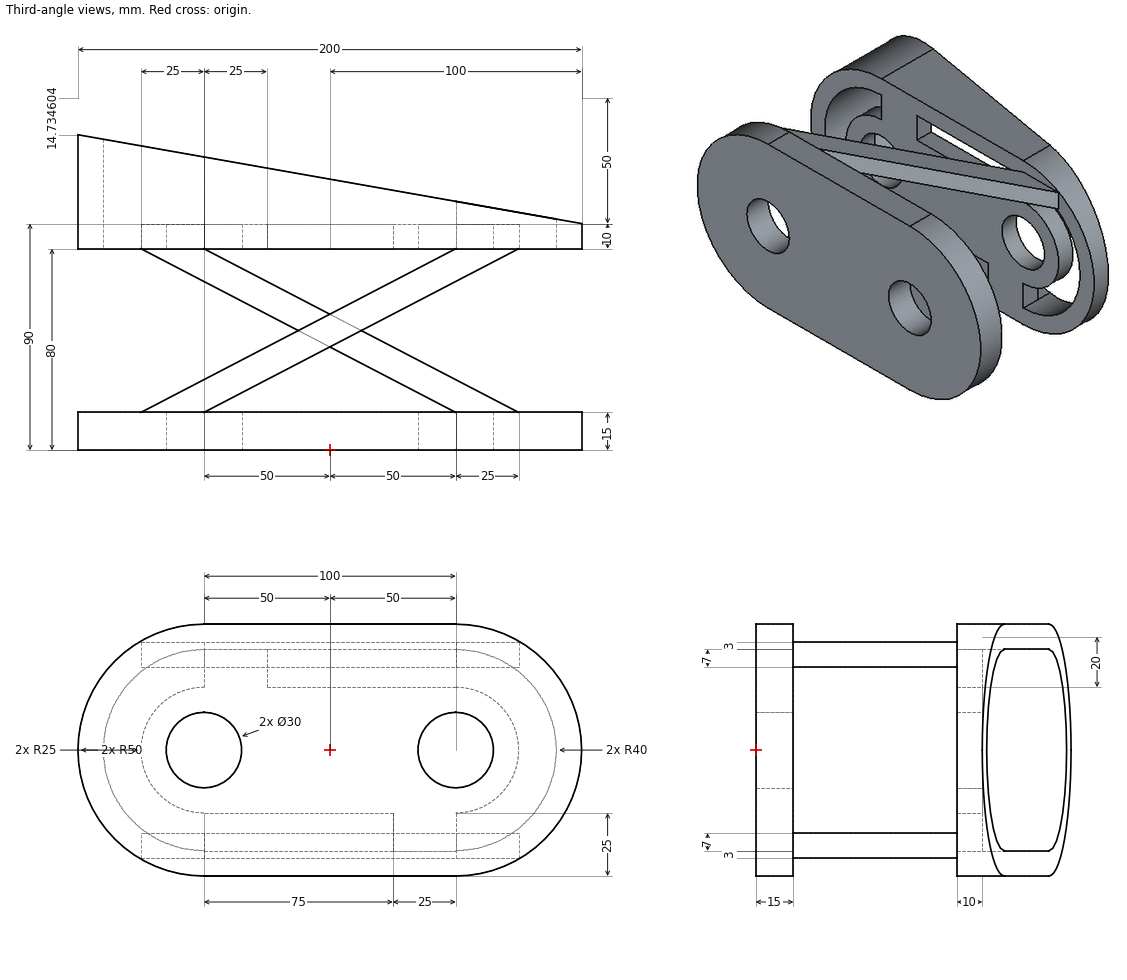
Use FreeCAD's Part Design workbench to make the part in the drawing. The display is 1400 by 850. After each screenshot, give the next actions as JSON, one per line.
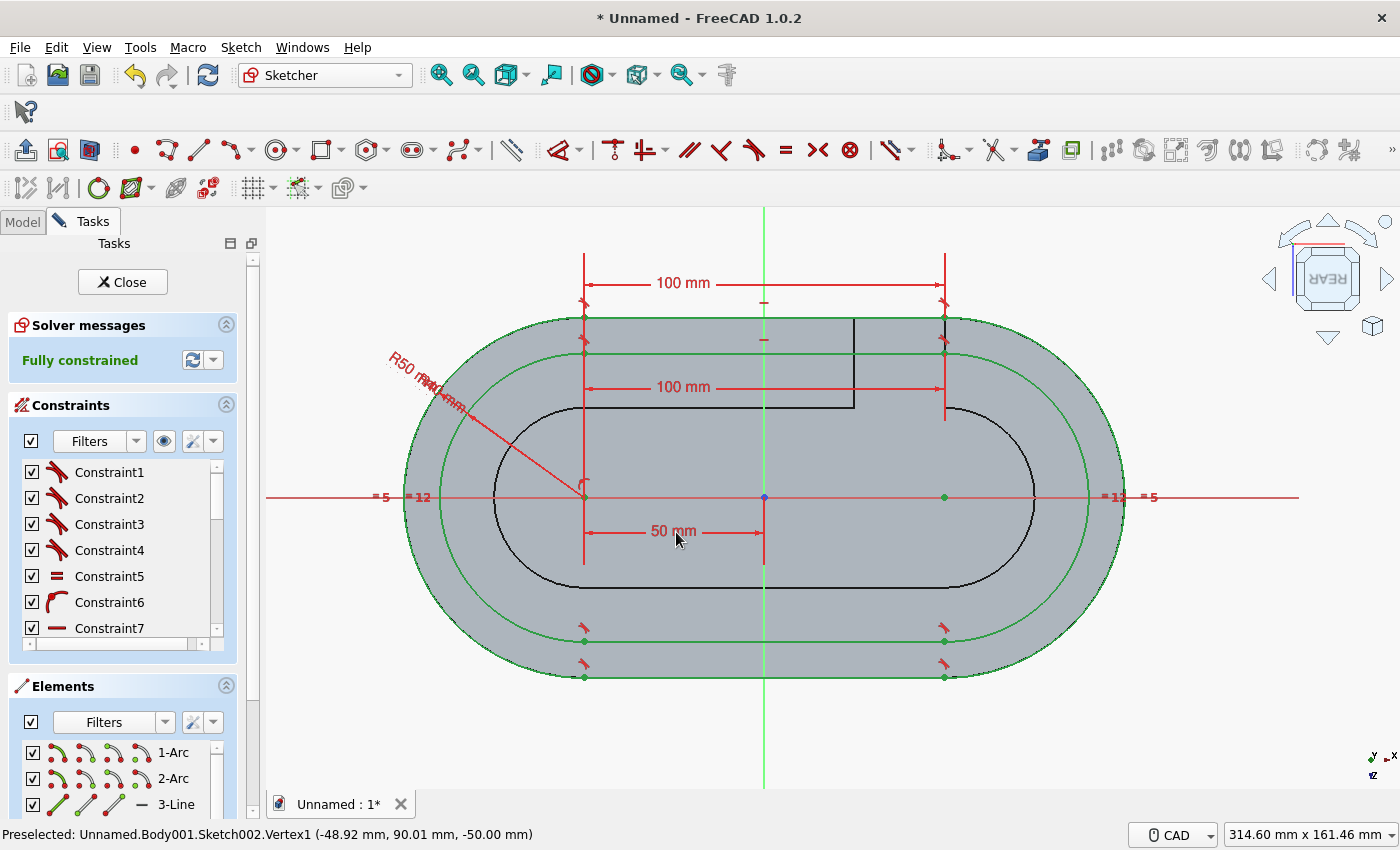
{"action": "left_click", "coordinate": [123, 282]}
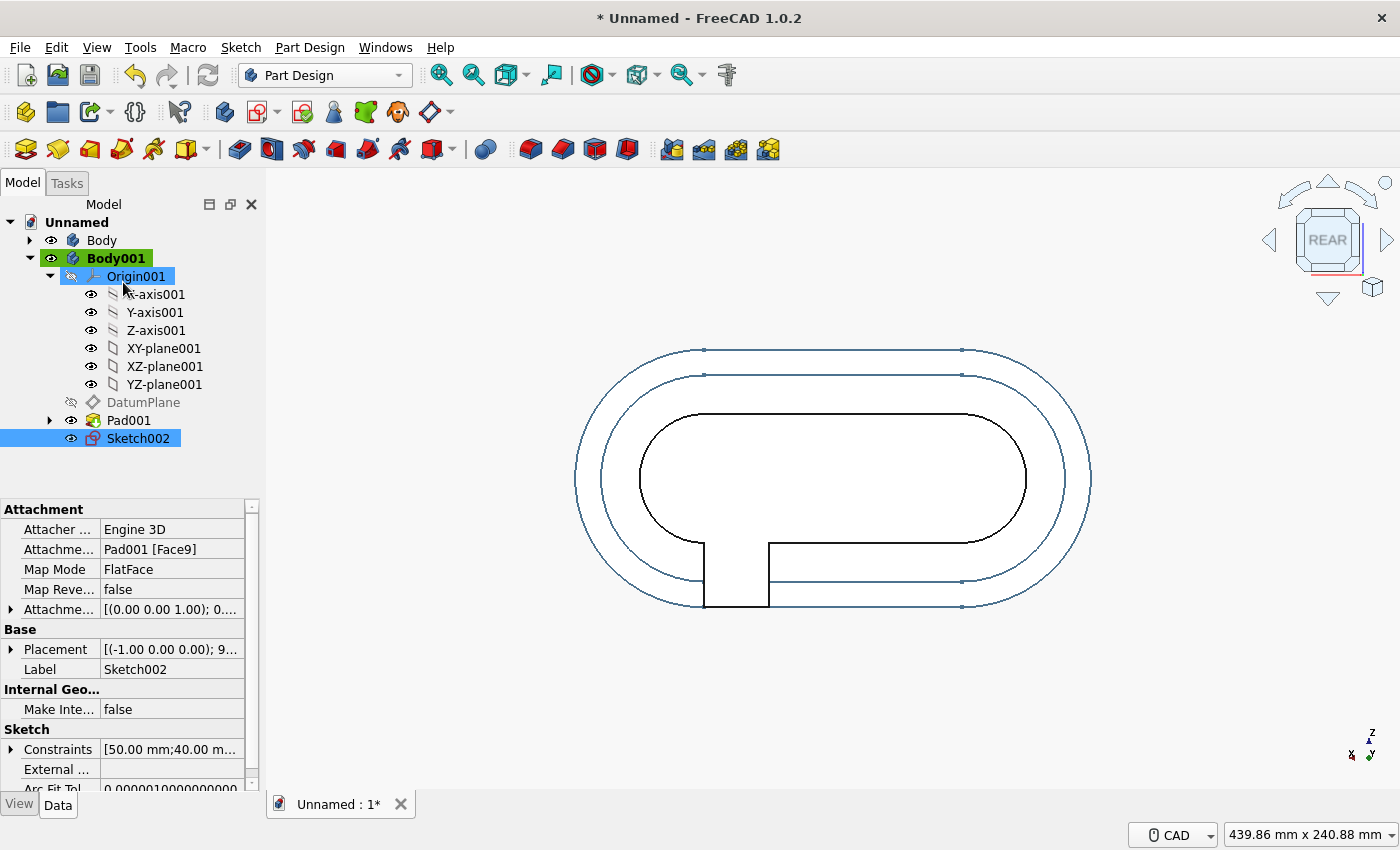
{"action": "left_click", "coordinate": [26, 150]}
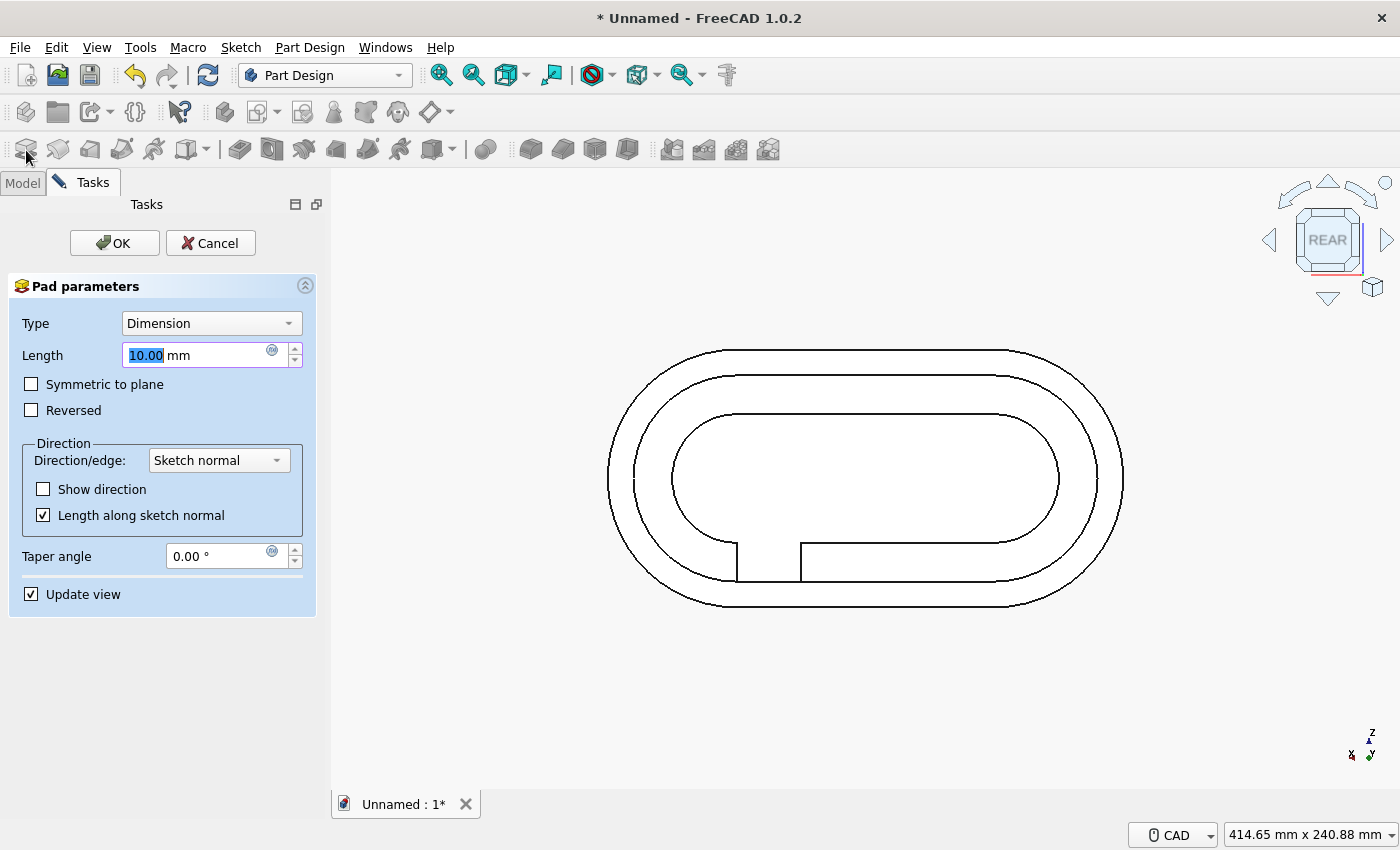
{"action": "left_click", "coordinate": [212, 324]}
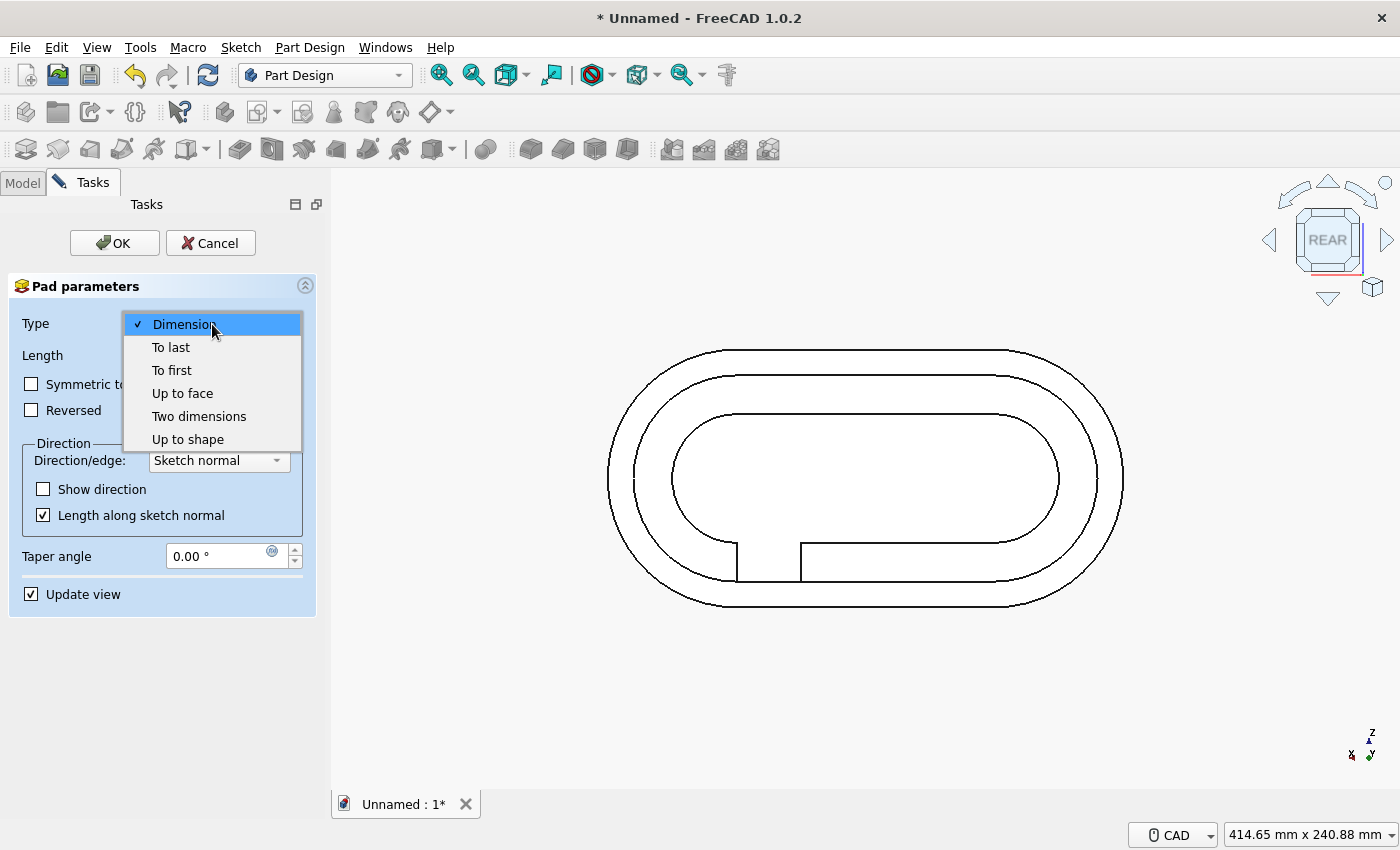
{"action": "left_click", "coordinate": [212, 416]}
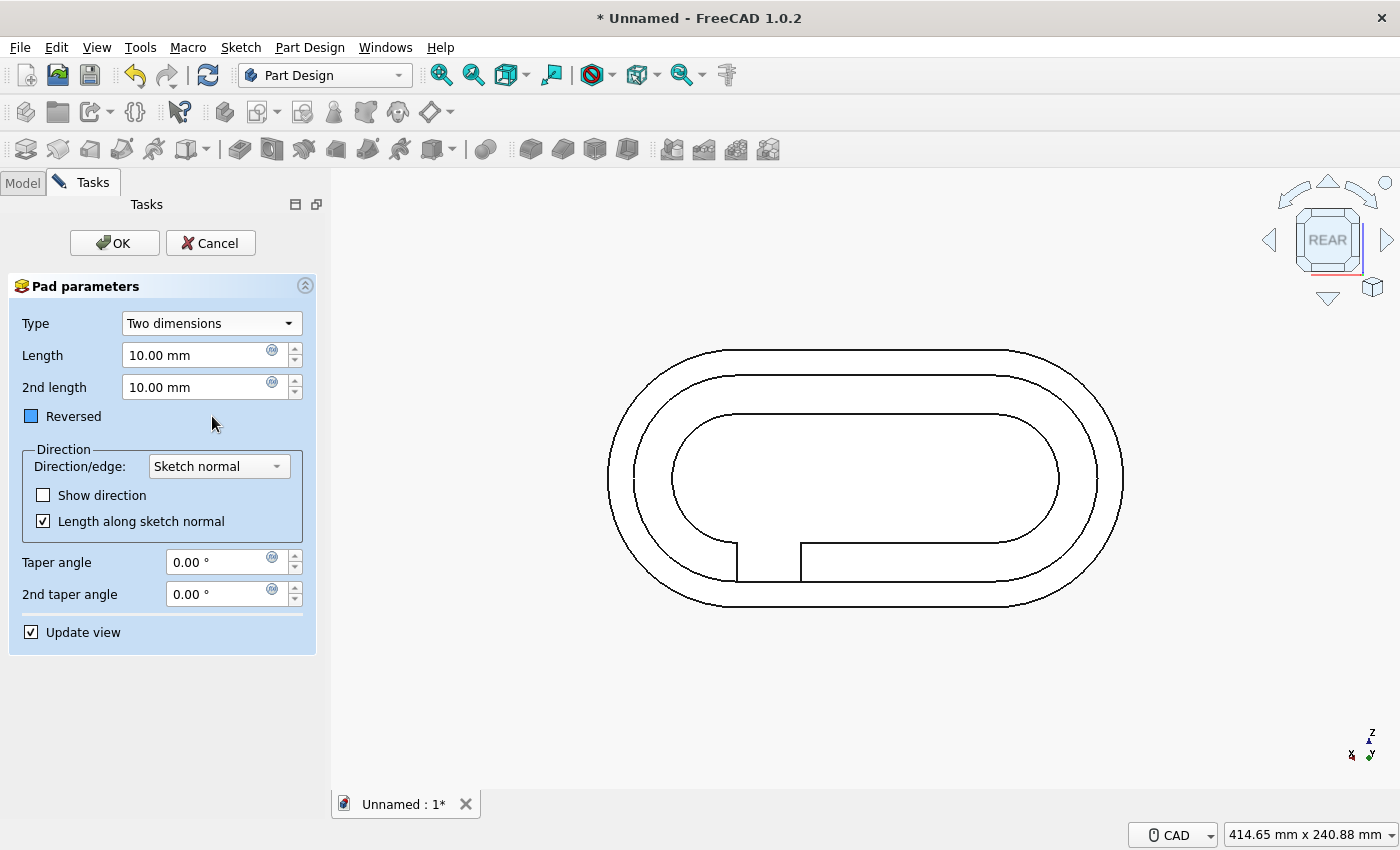
{"action": "triple_click", "coordinate": [204, 355]}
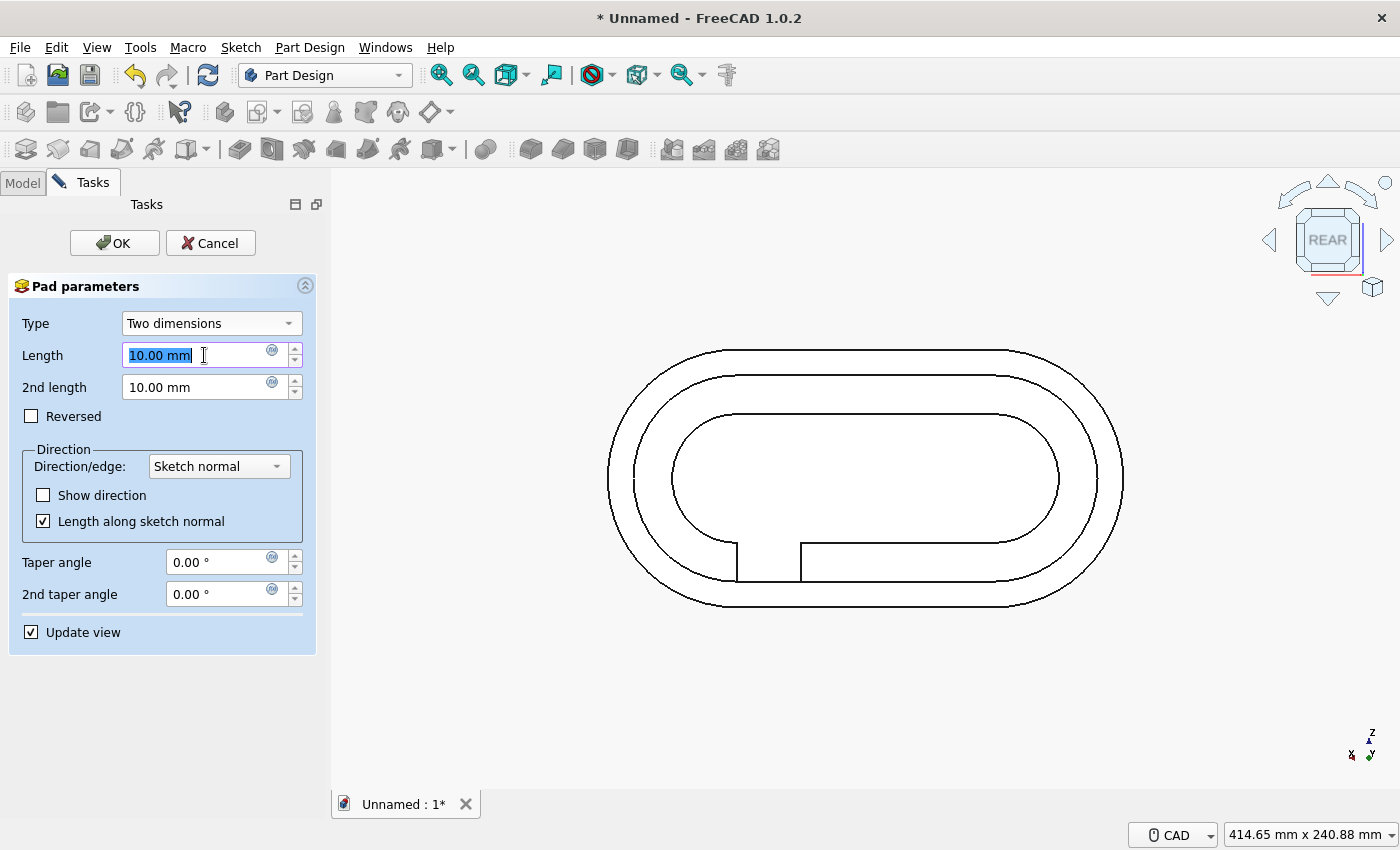
{"action": "type", "text": "50"}
{"action": "key", "text": "Tab"}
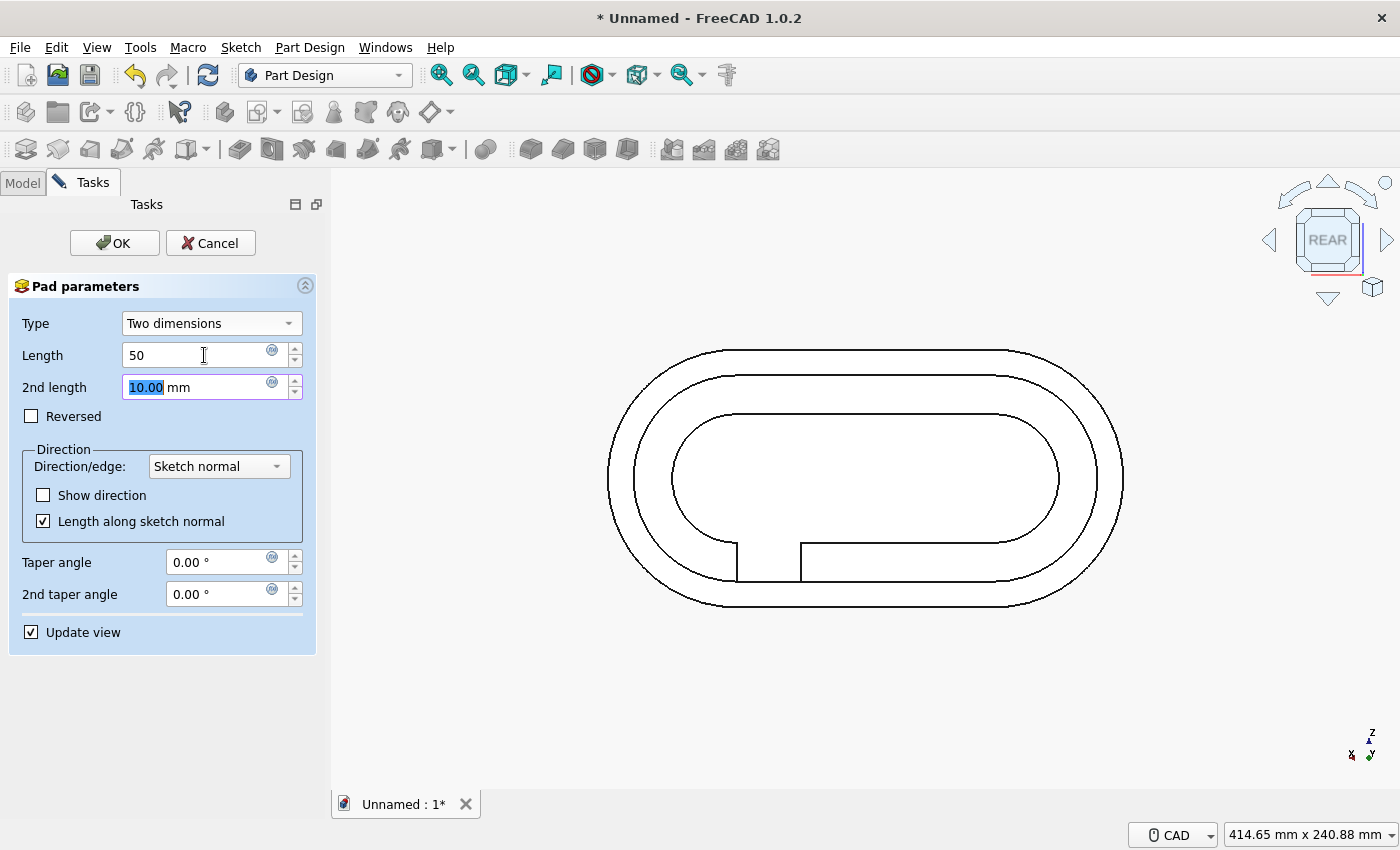
{"action": "type", "text": "10"}
{"action": "key", "text": "Tab"}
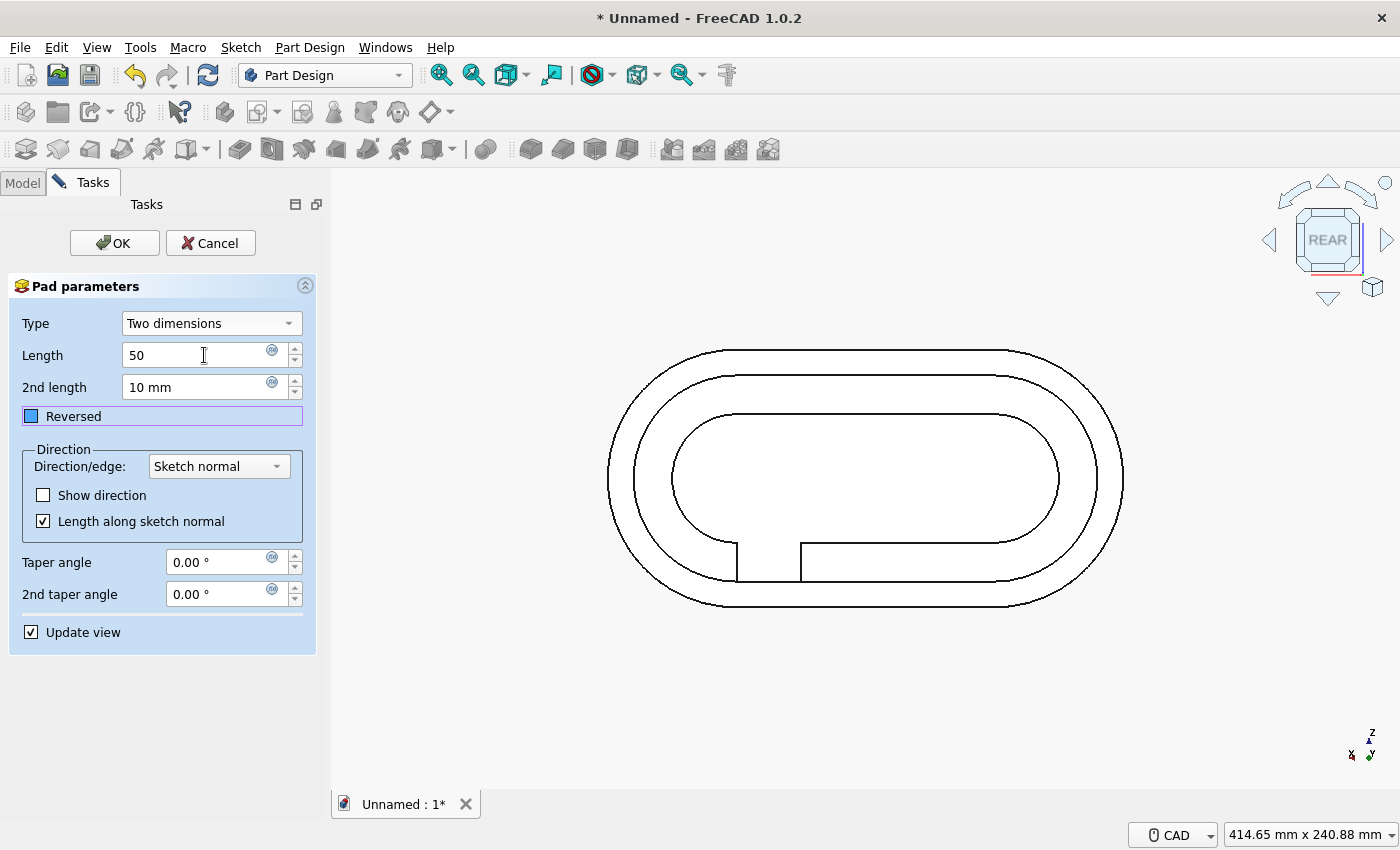
{"action": "left_click", "coordinate": [115, 243]}